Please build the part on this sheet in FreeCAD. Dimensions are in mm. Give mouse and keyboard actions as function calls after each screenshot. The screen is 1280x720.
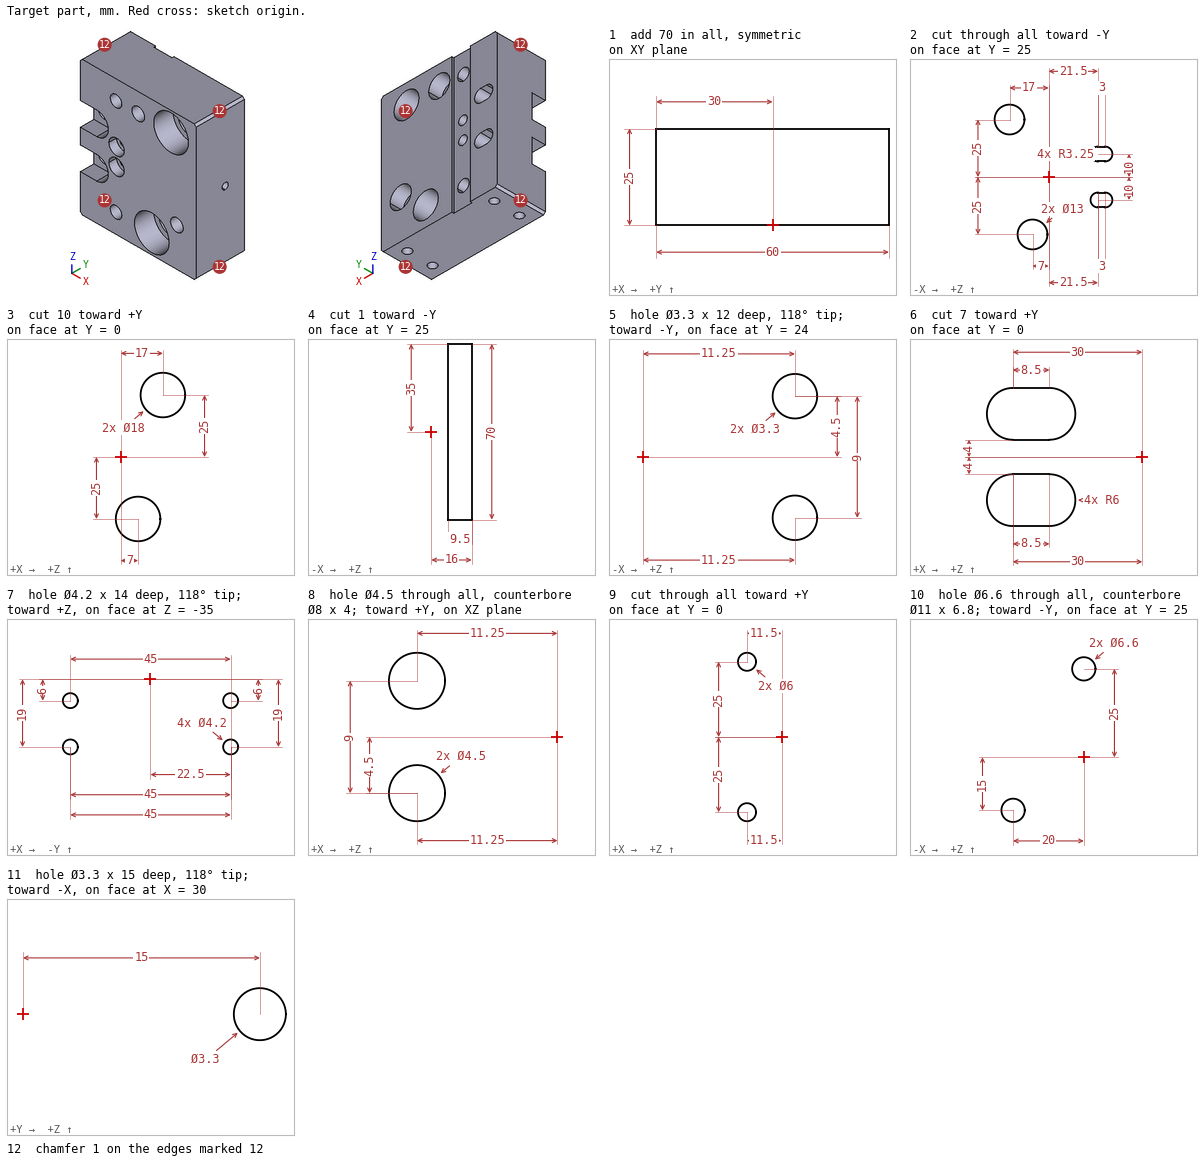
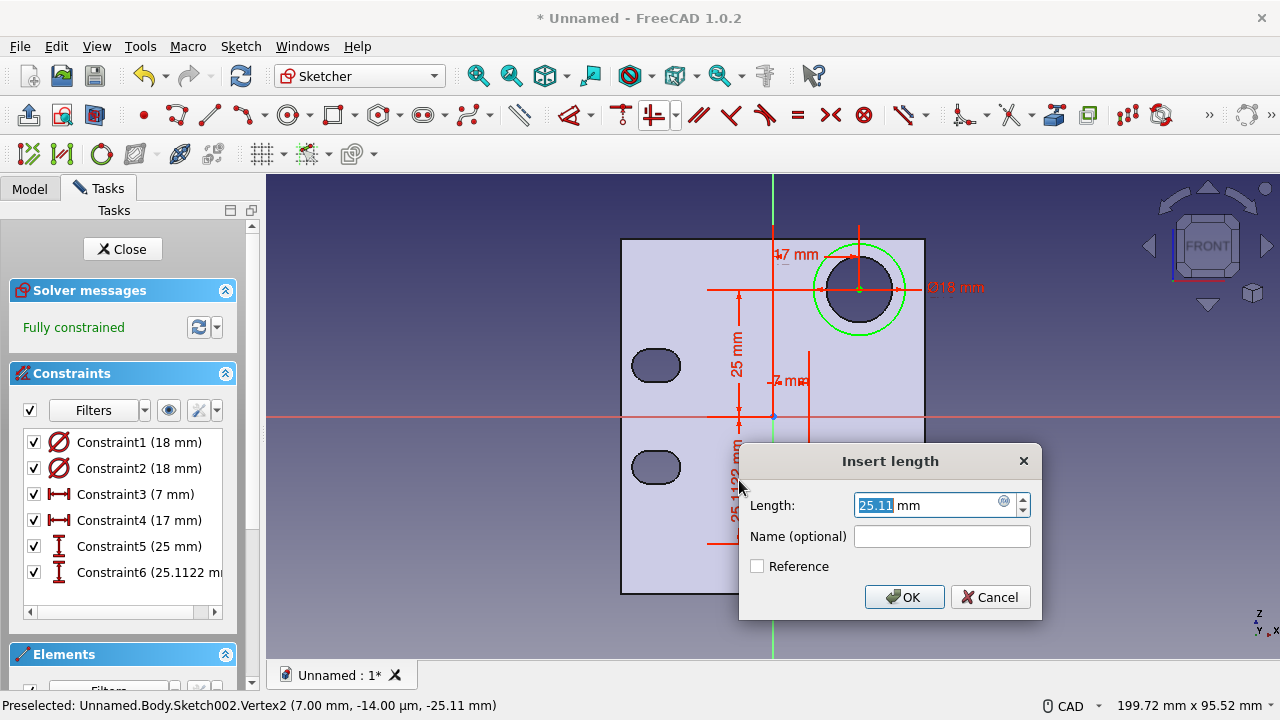
text(25)
key(Return)
key(Escape)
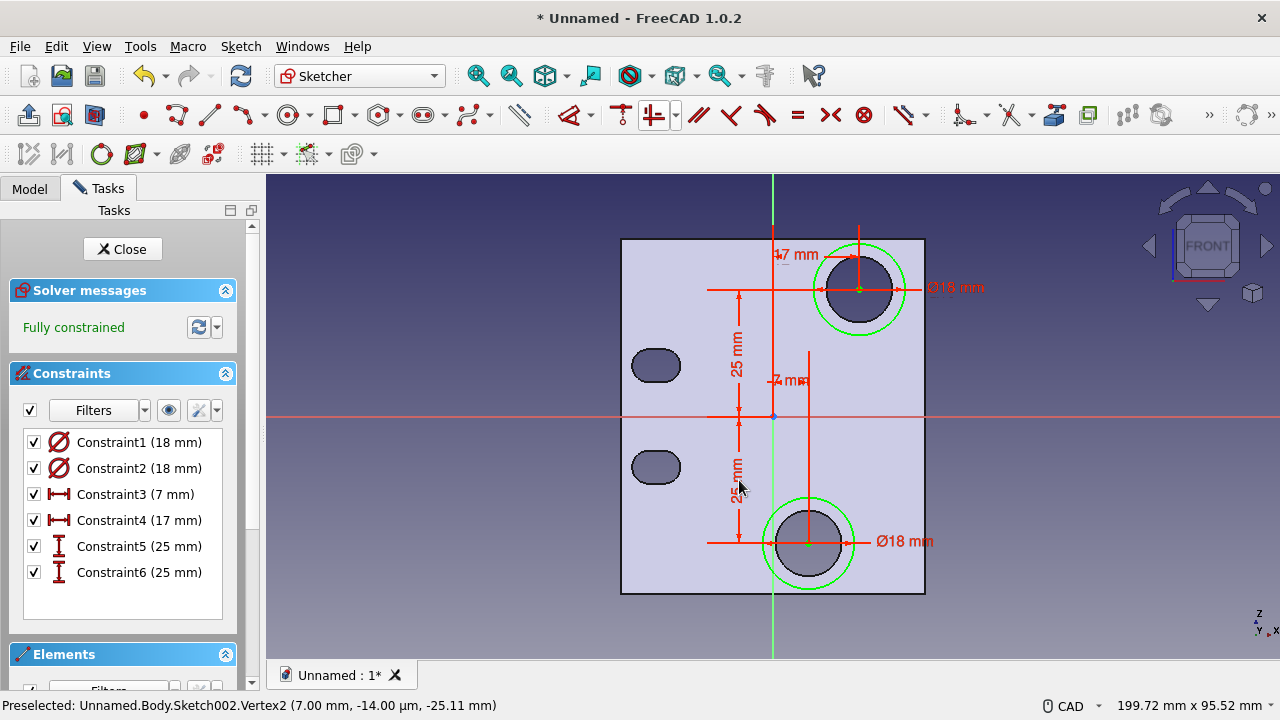
click(123, 249)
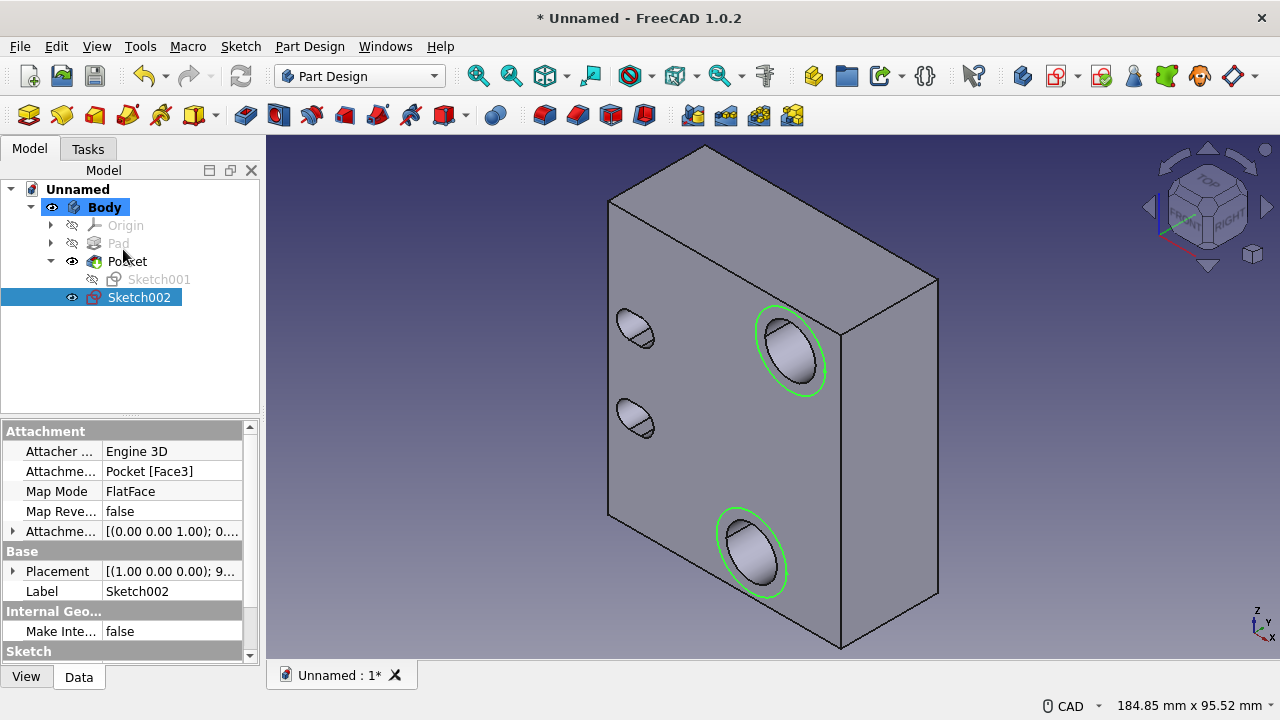
click(246, 116)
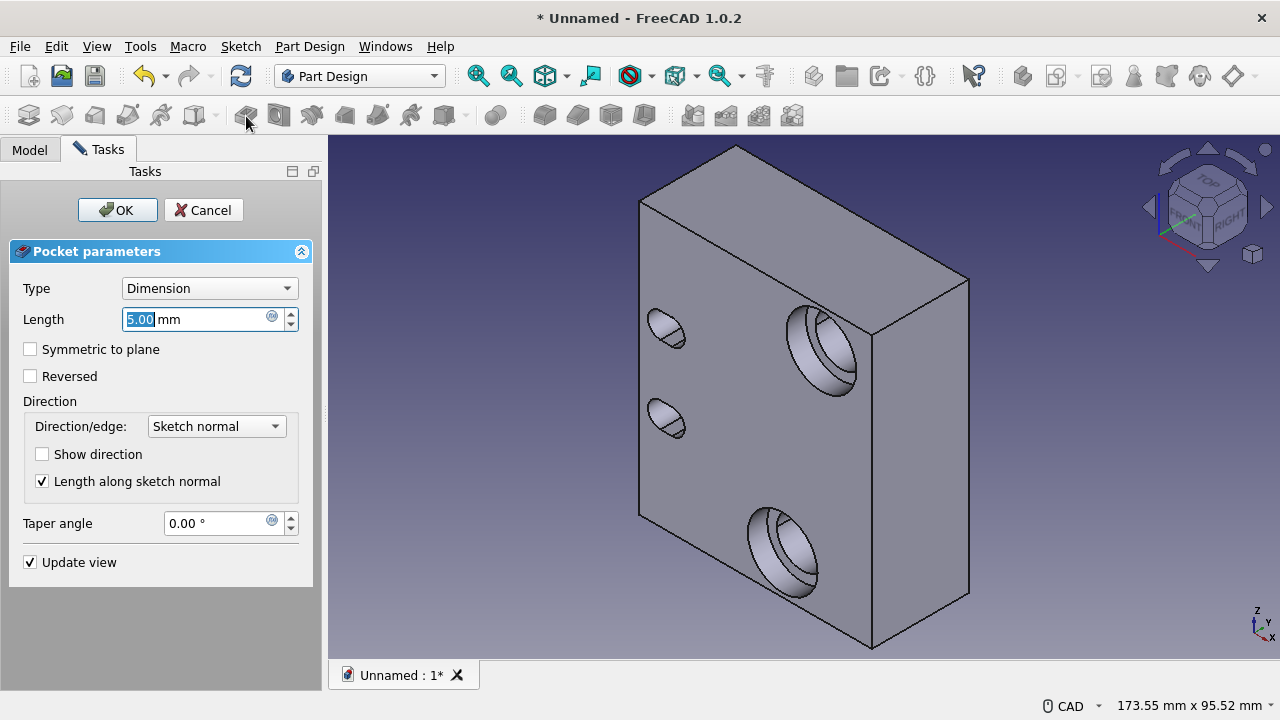
text(10)
key(Tab)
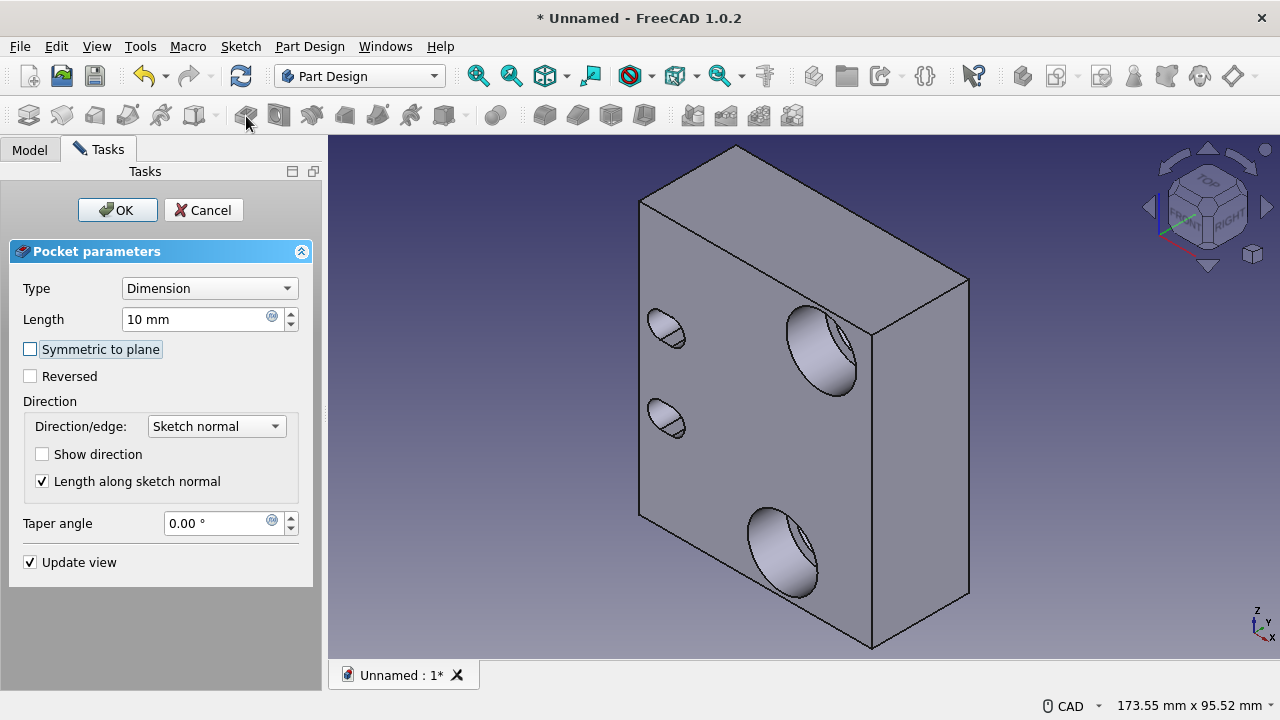
click(118, 210)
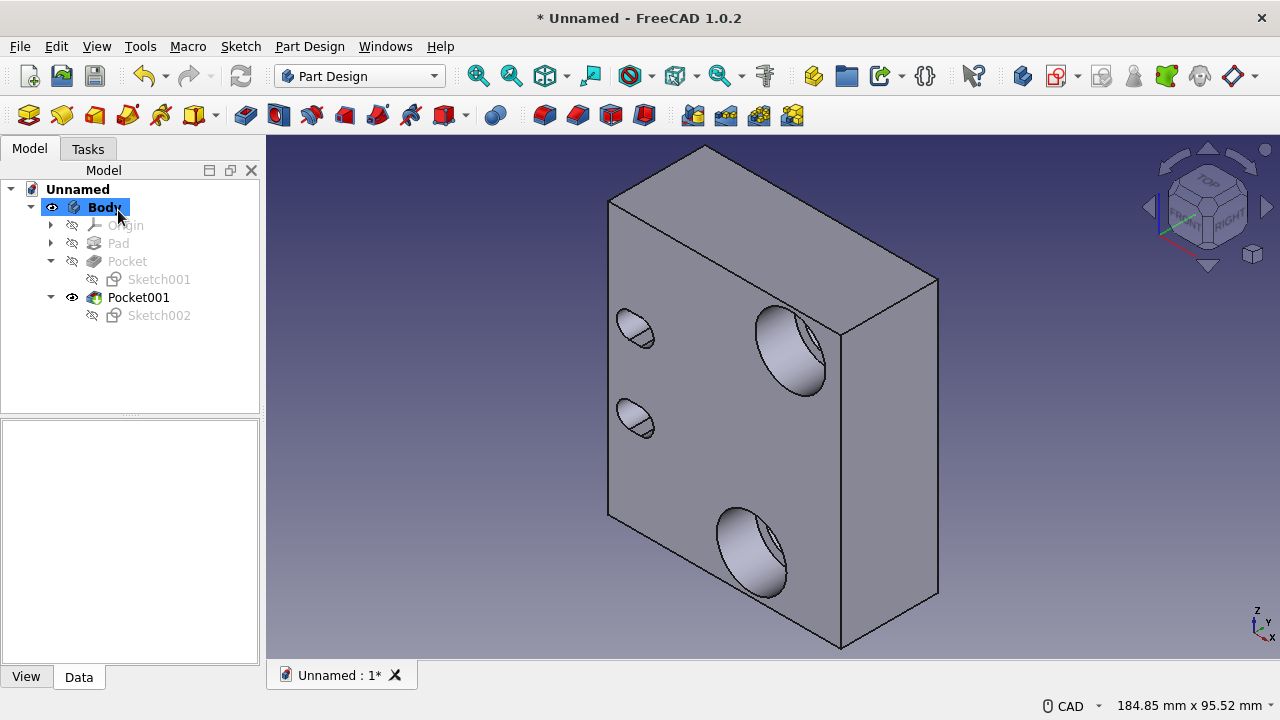
key(4)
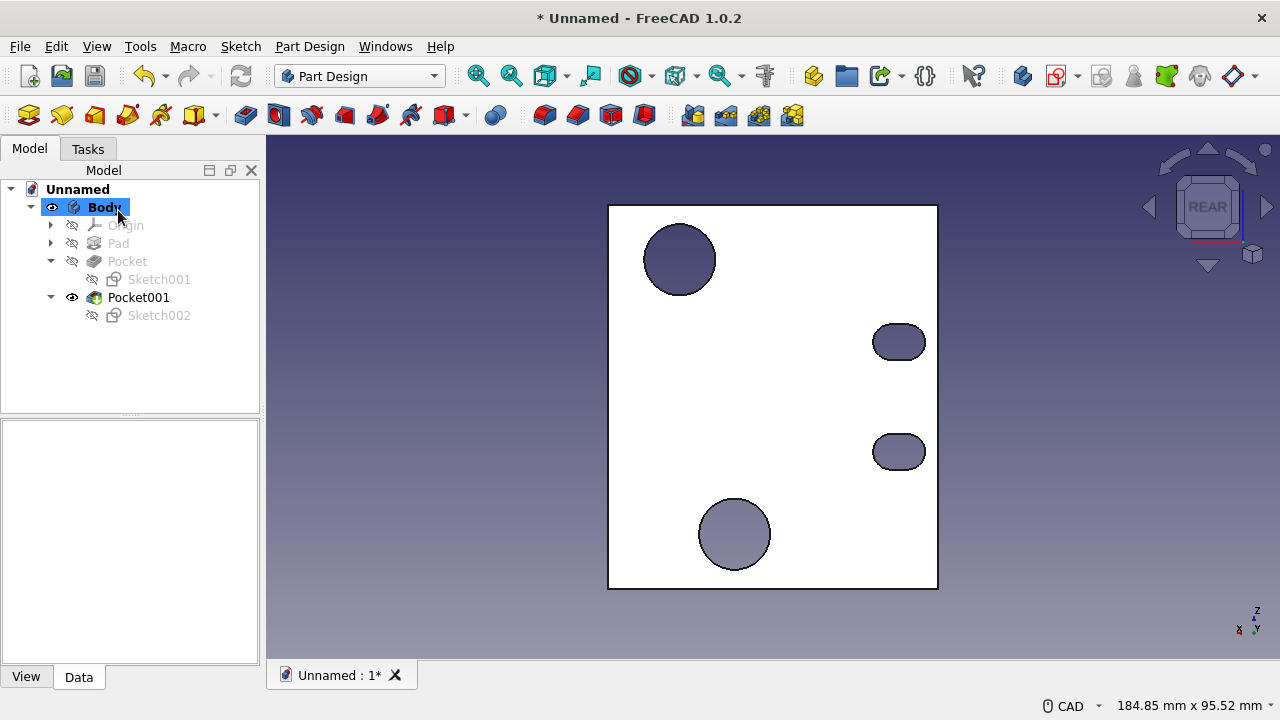
click(773, 396)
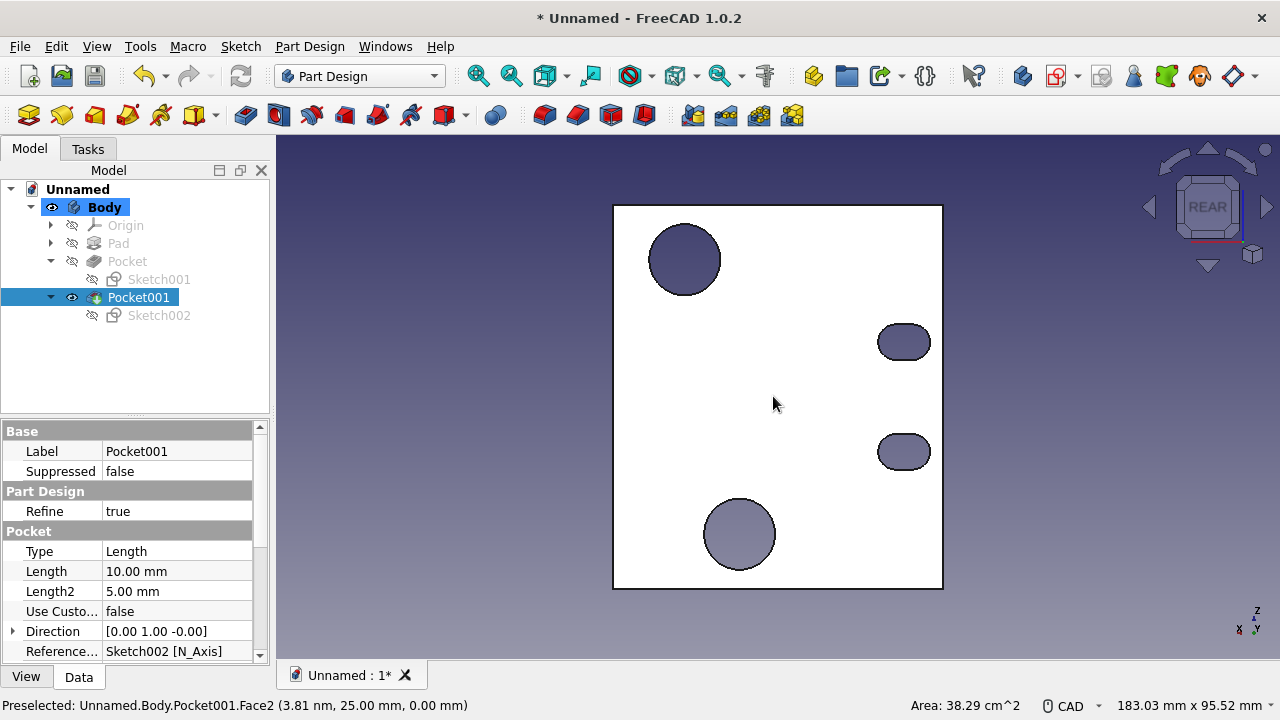
click(1056, 76)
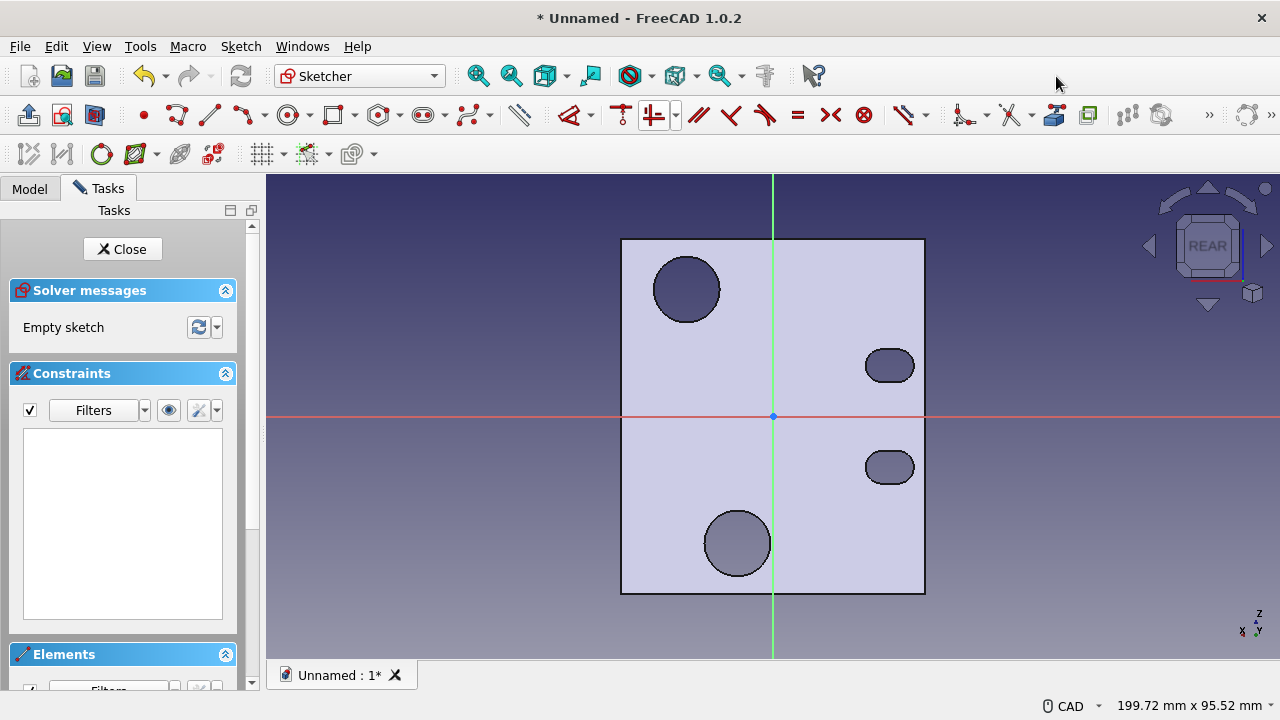
key(g)
key(r)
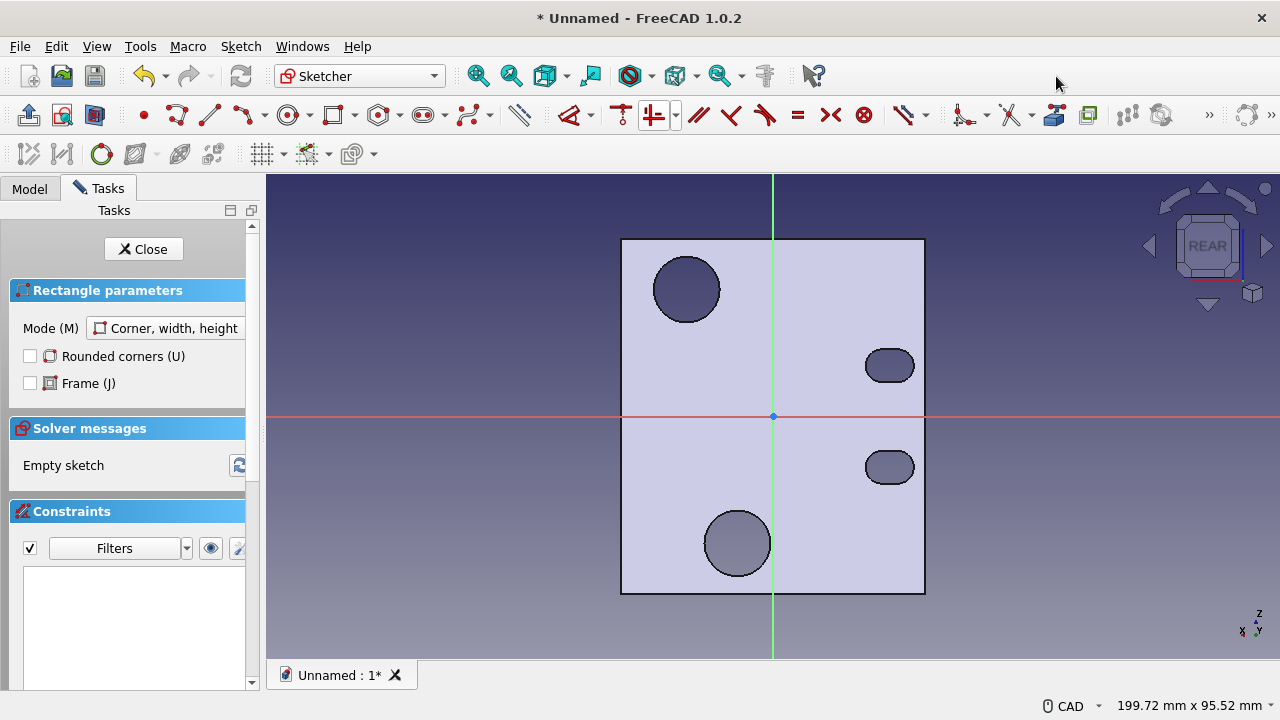
click(806, 239)
move(854, 594)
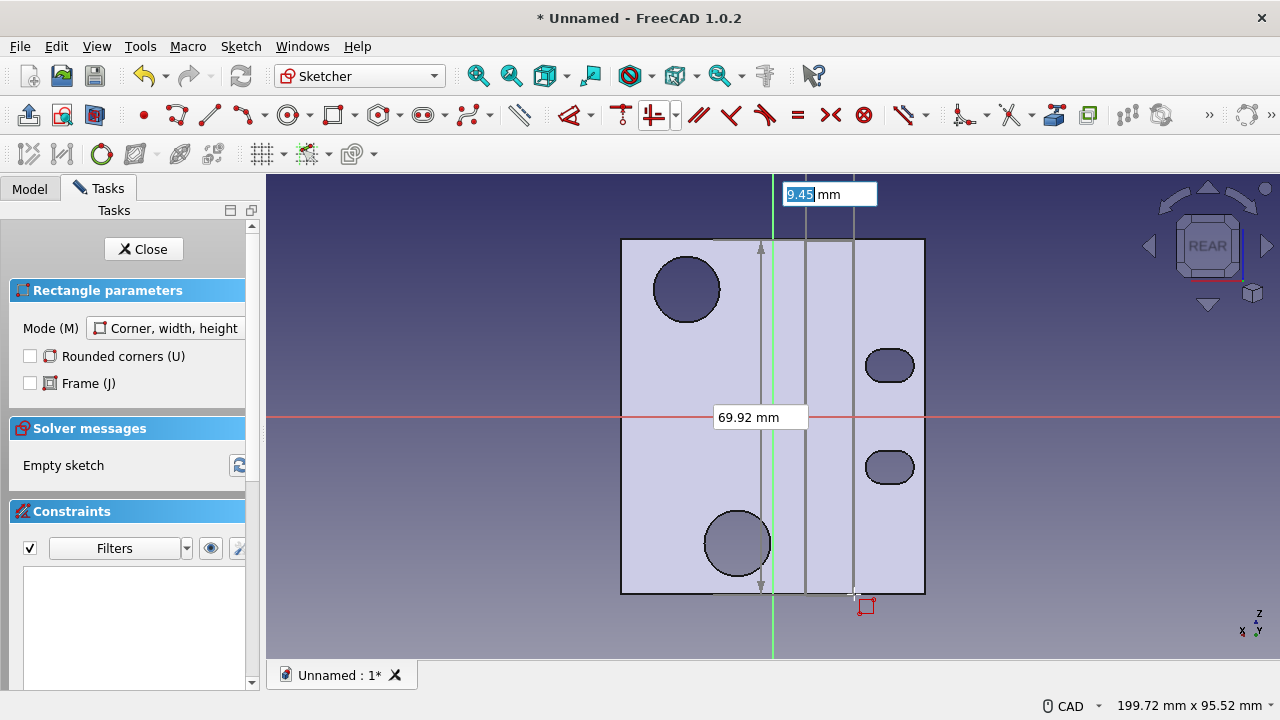
text(9.5)
key(Tab)
text(70)
key(Return)
key(Escape)